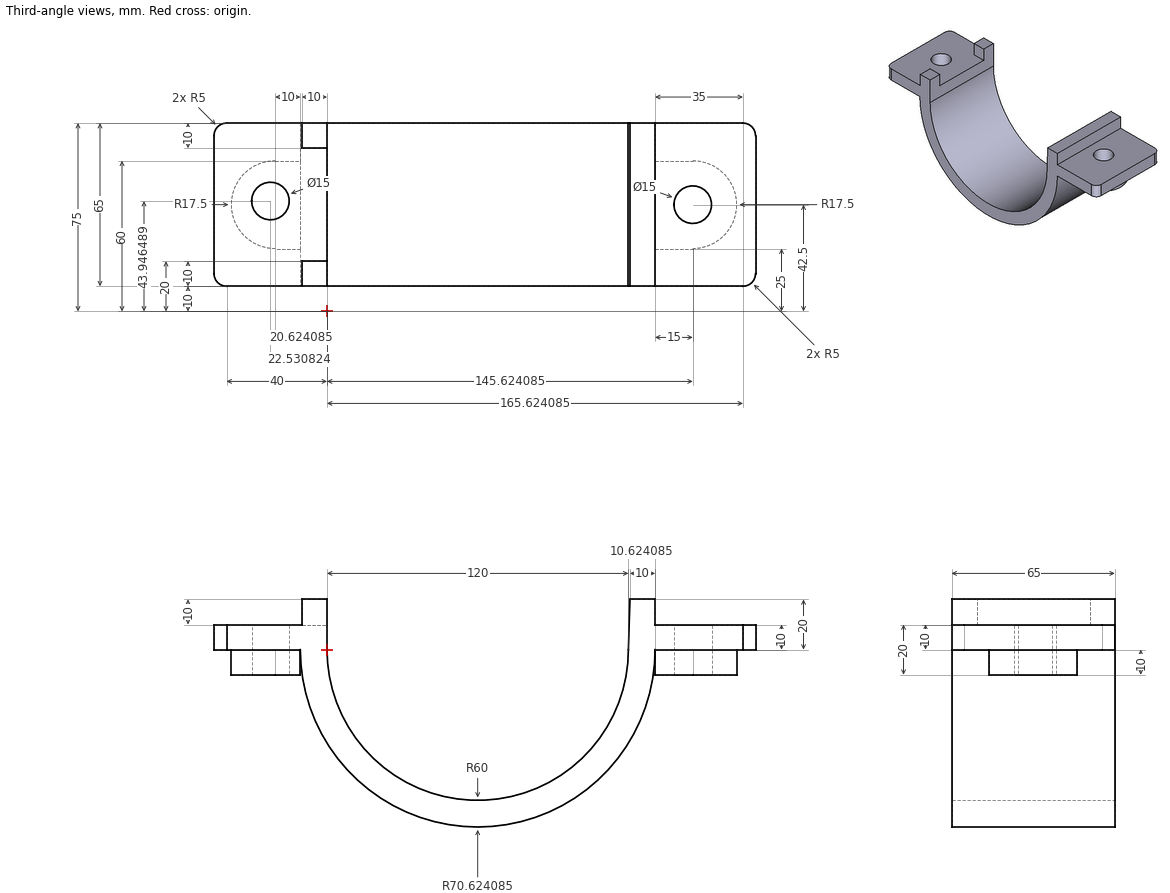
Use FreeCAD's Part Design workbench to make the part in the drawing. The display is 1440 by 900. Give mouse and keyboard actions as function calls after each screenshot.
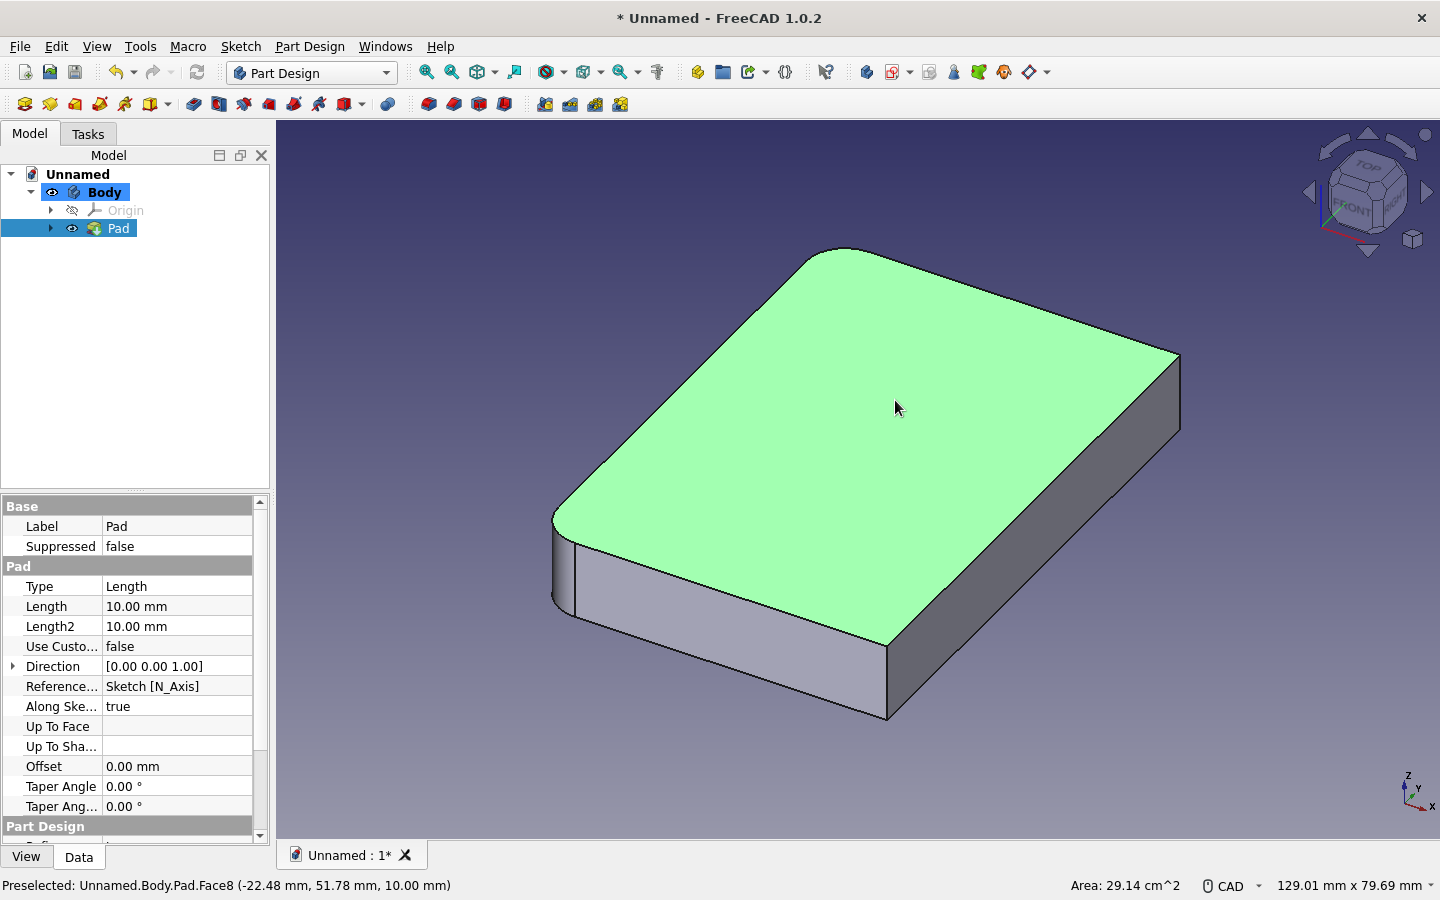
click(892, 72)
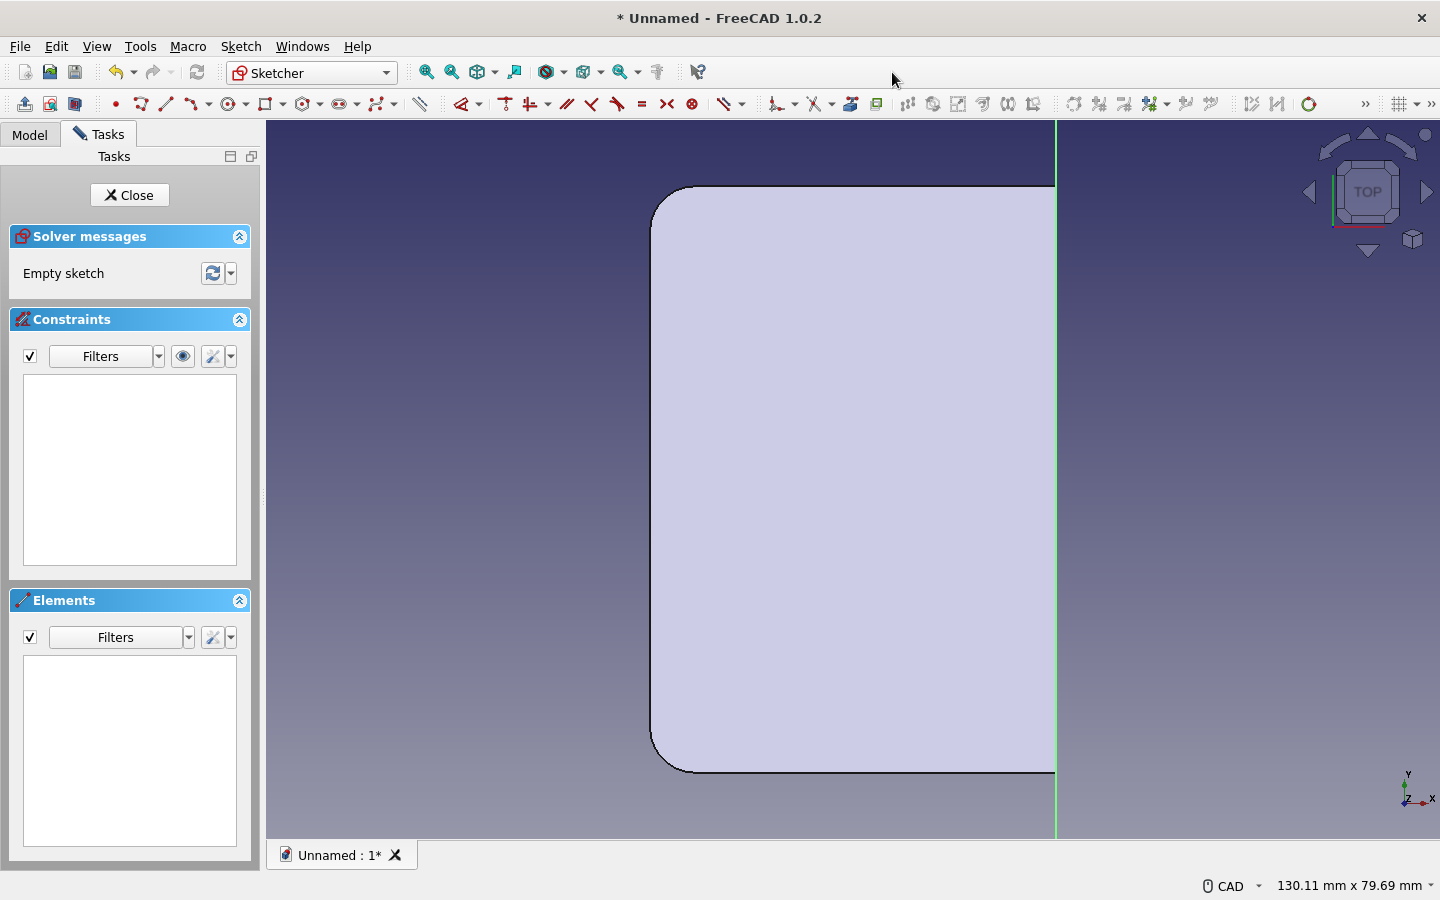
scroll(324, 388, down, 2)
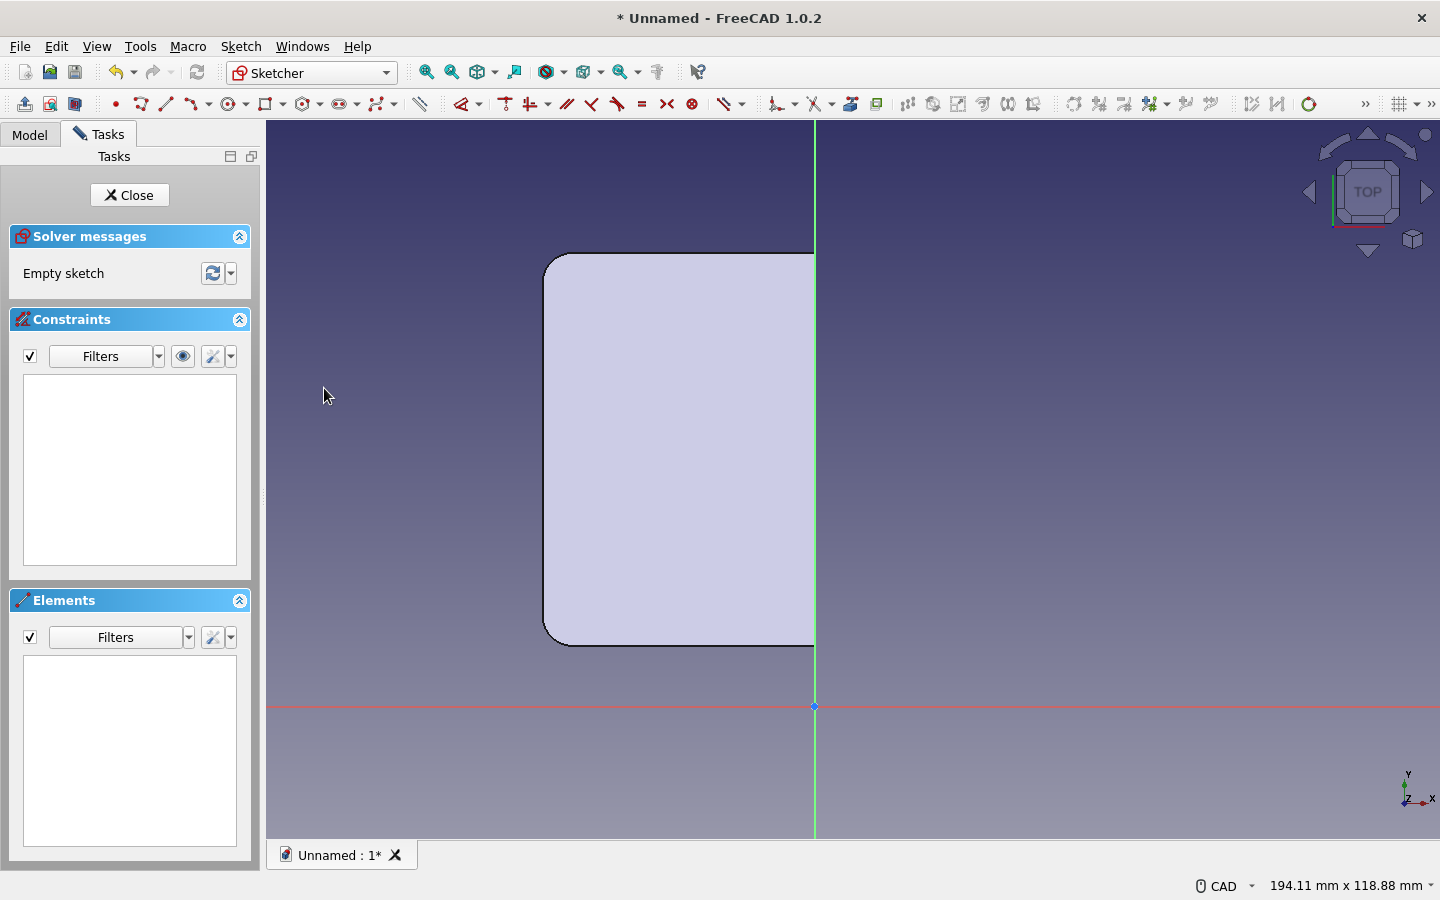
key(g)
key(r)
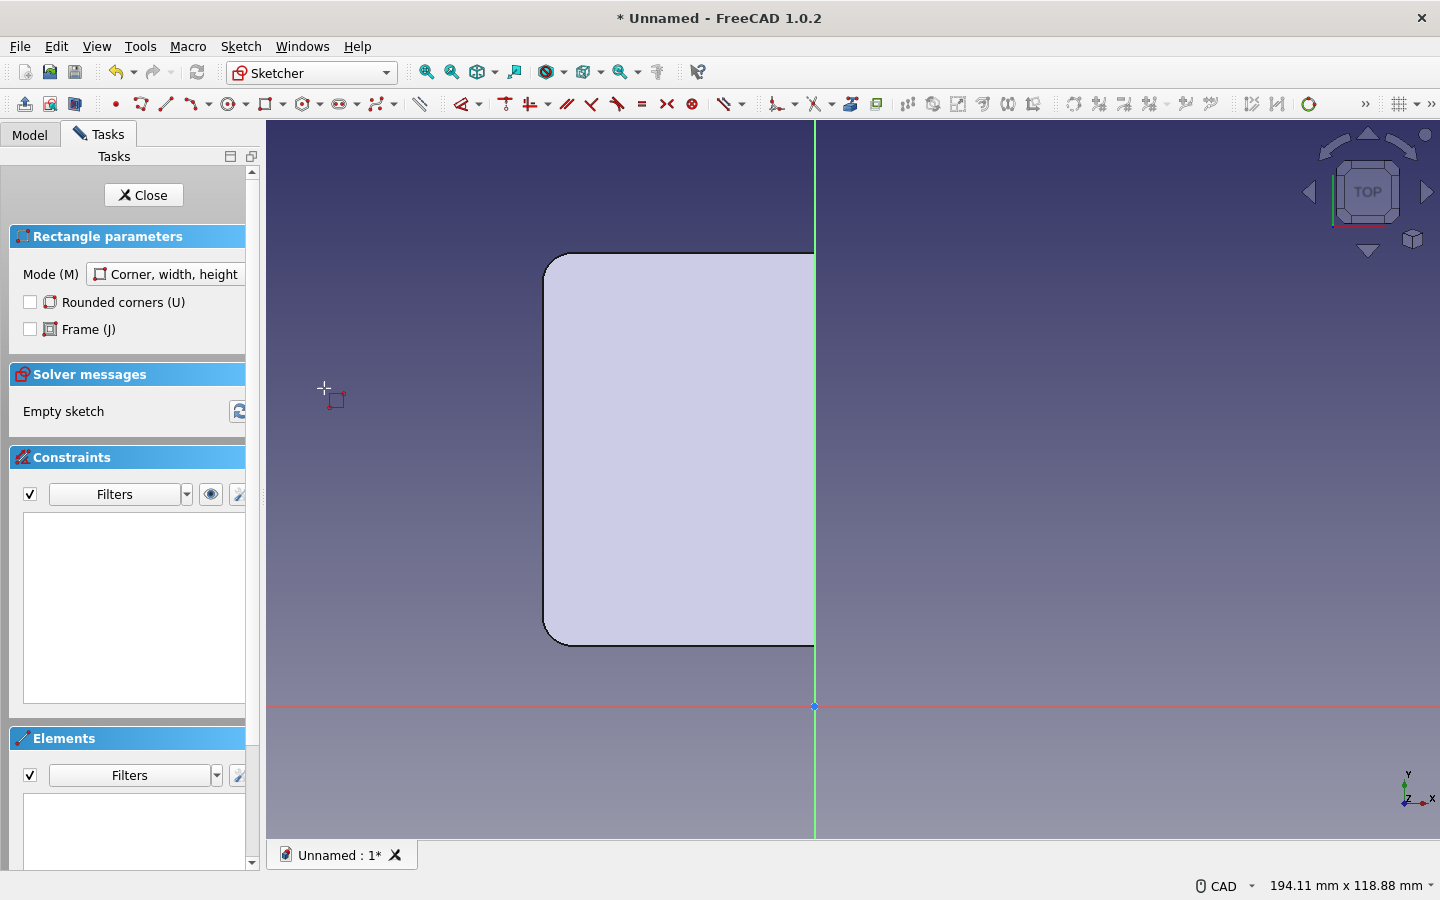
click(754, 253)
click(815, 313)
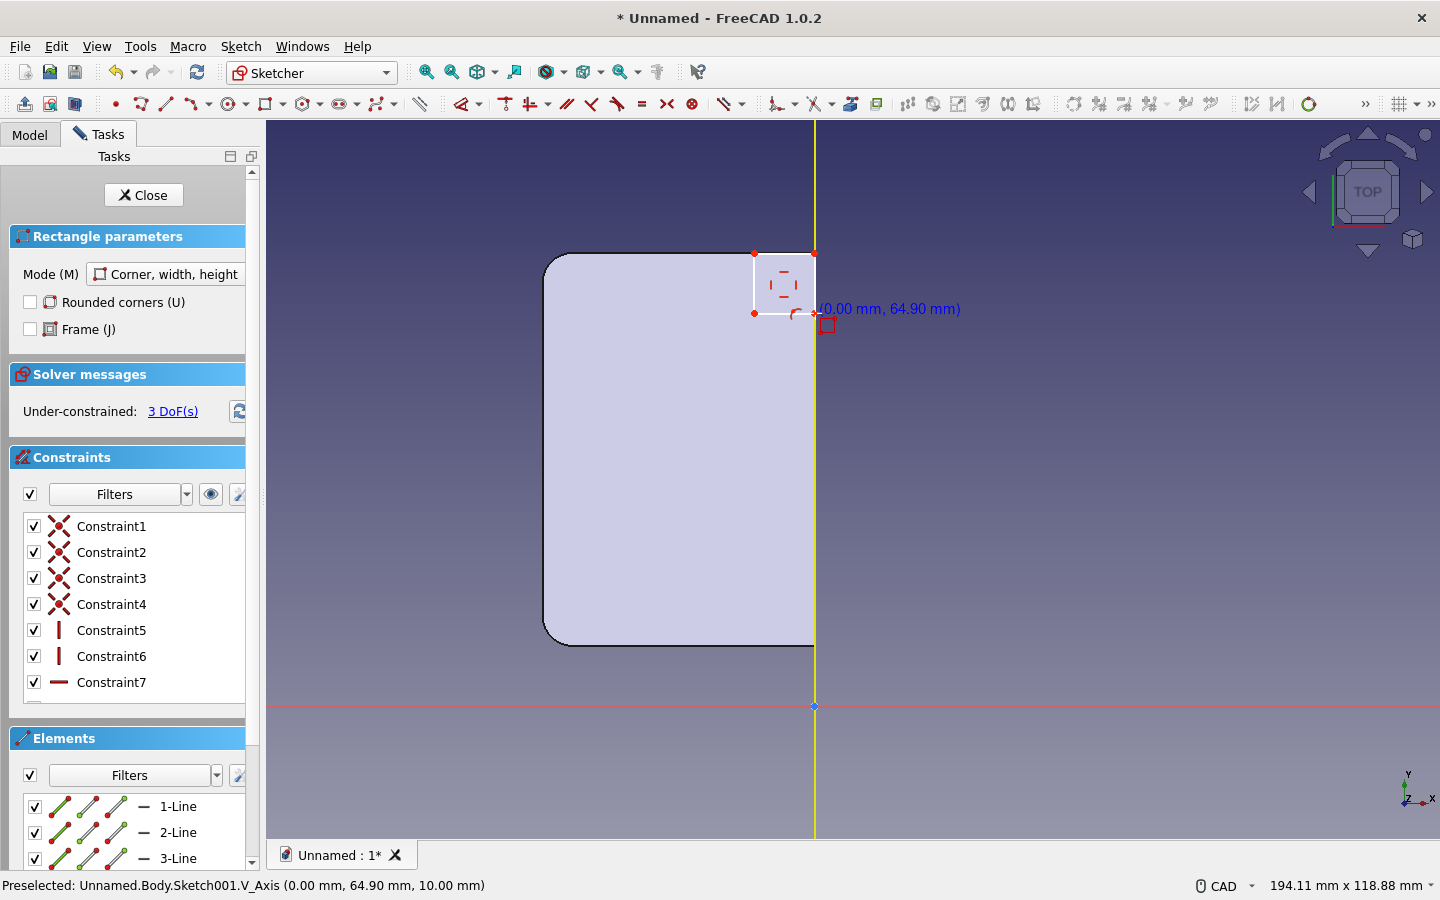
click(754, 586)
click(815, 646)
key(Escape)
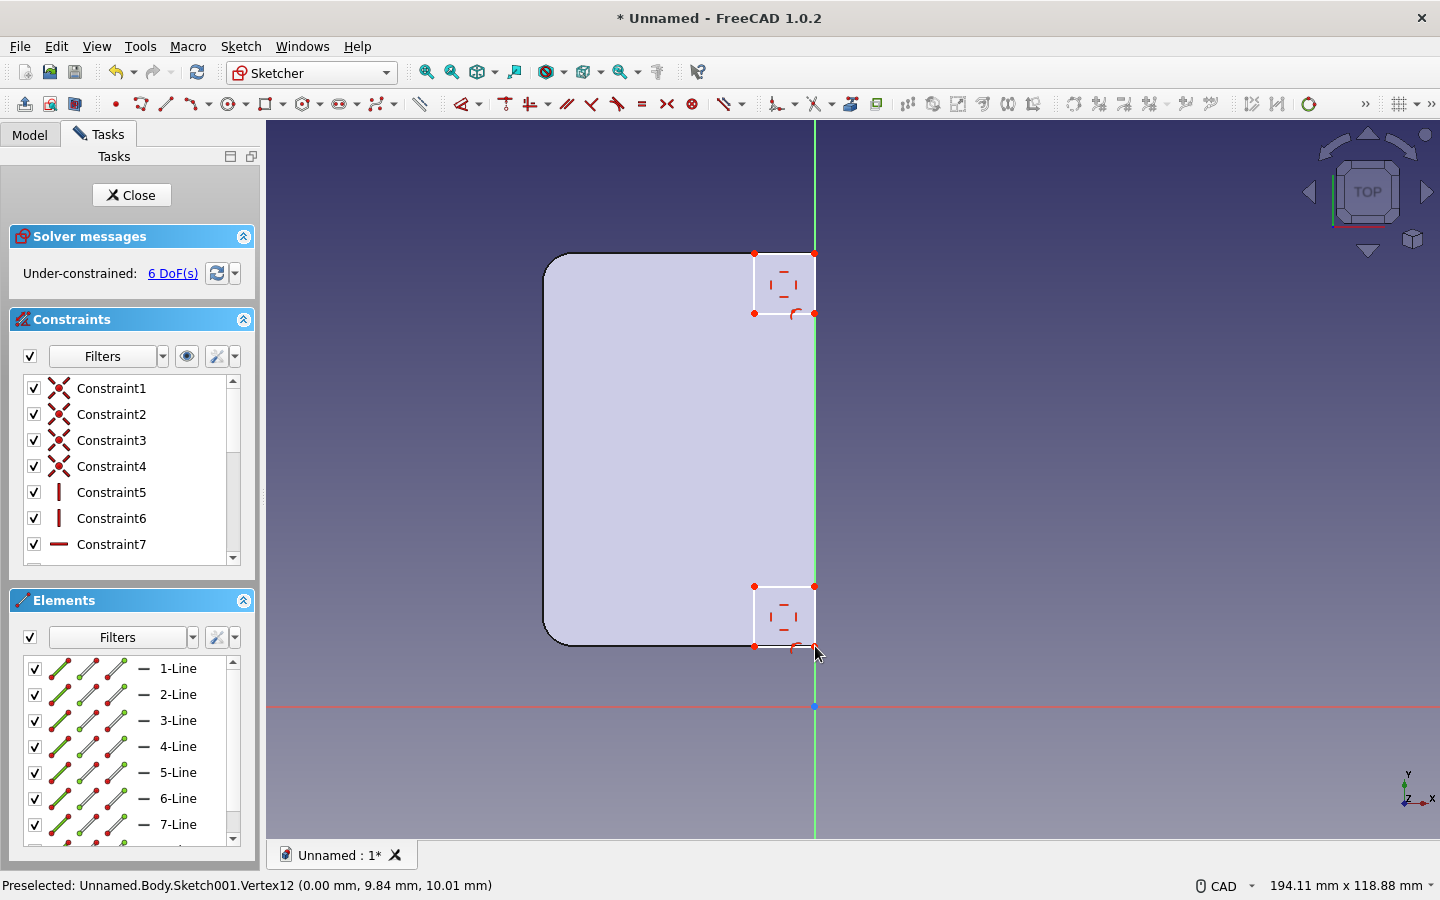
key(d)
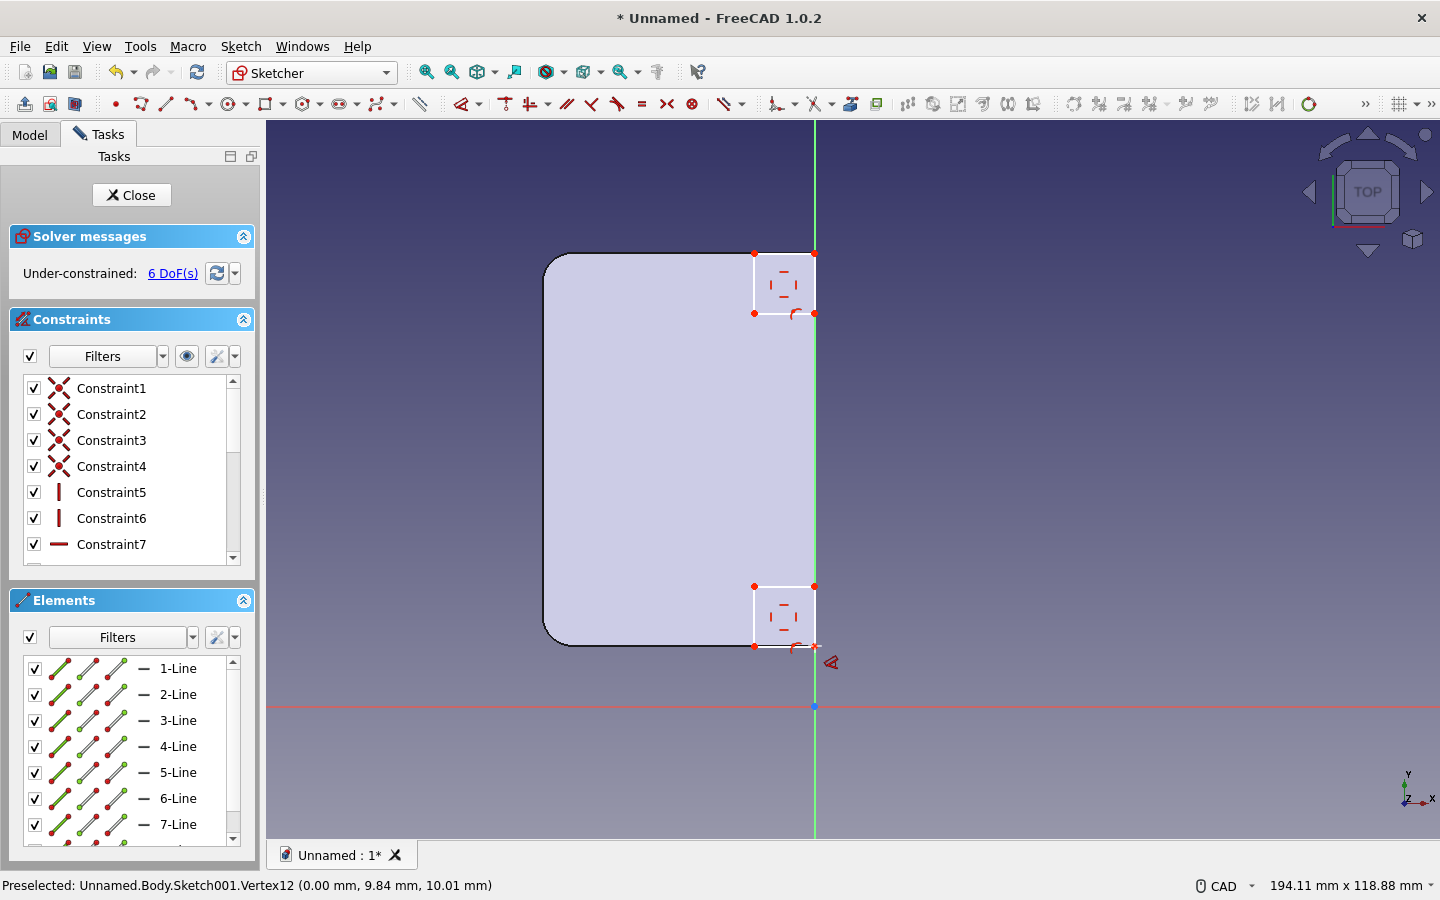
click(754, 272)
click(720, 284)